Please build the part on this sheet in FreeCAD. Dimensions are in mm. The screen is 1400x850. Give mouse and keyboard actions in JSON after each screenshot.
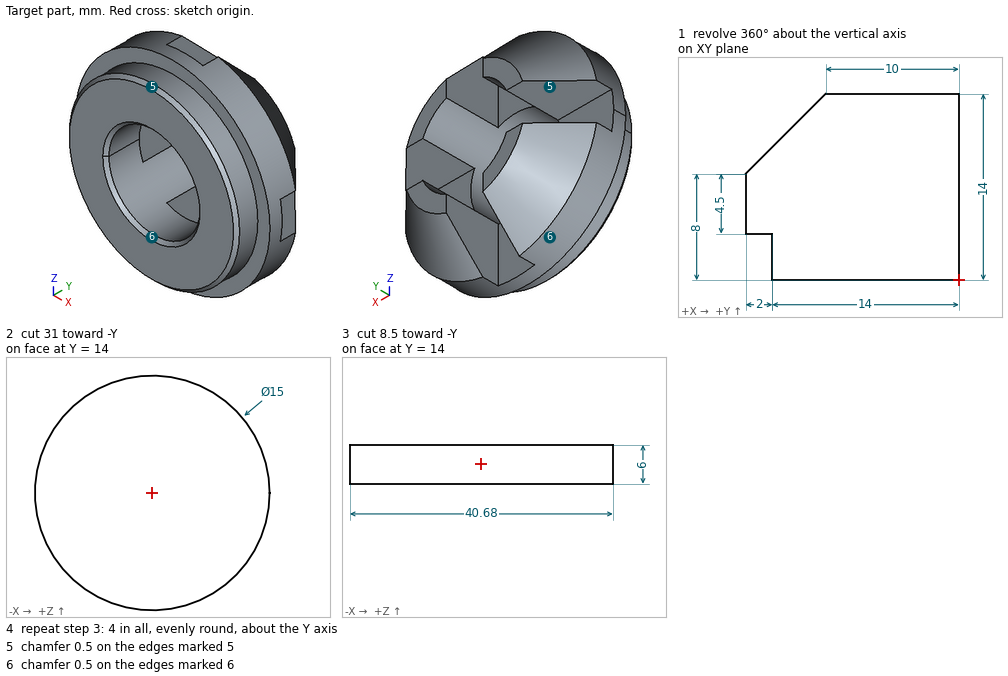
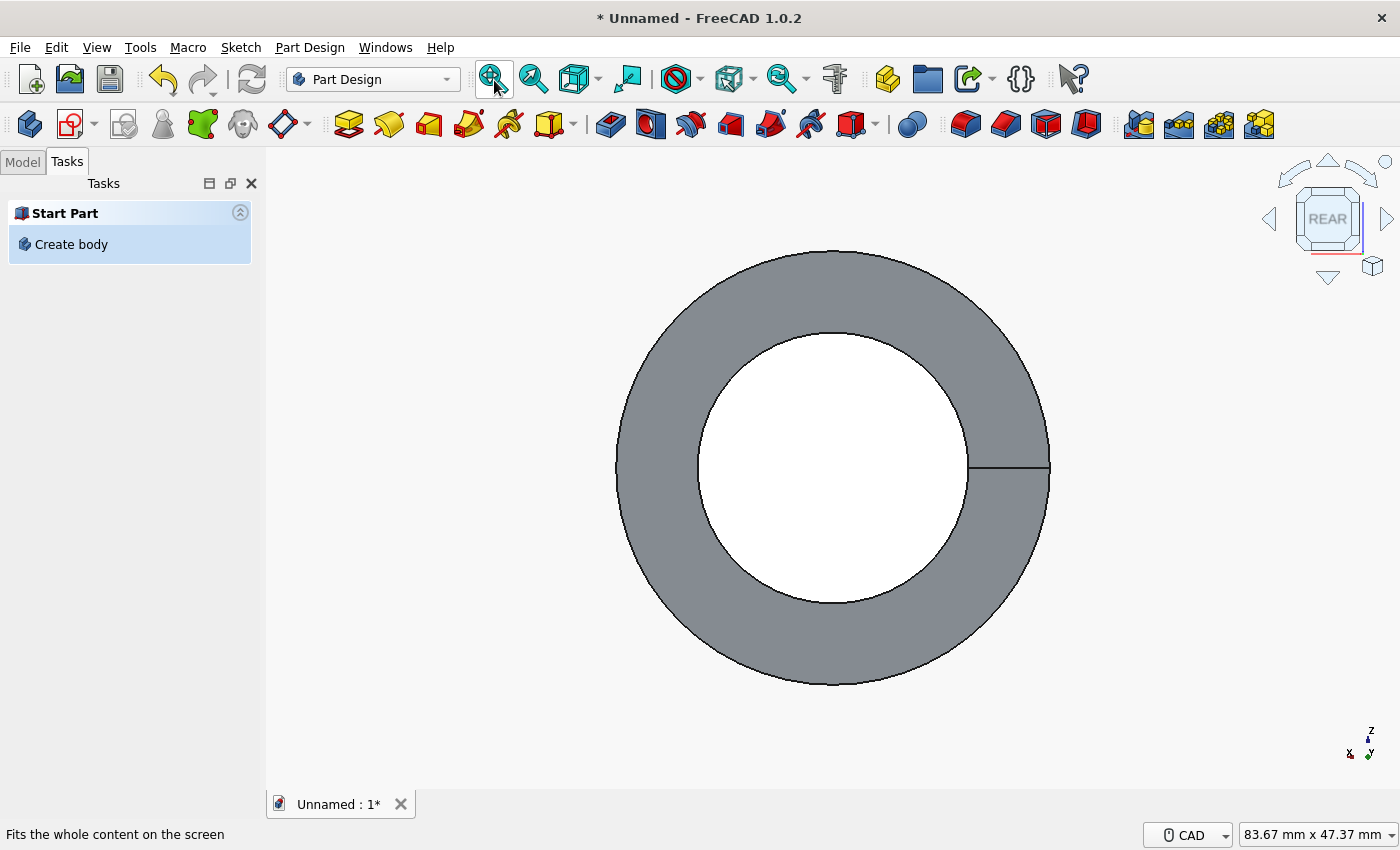
{"action": "left_click", "coordinate": [833, 467]}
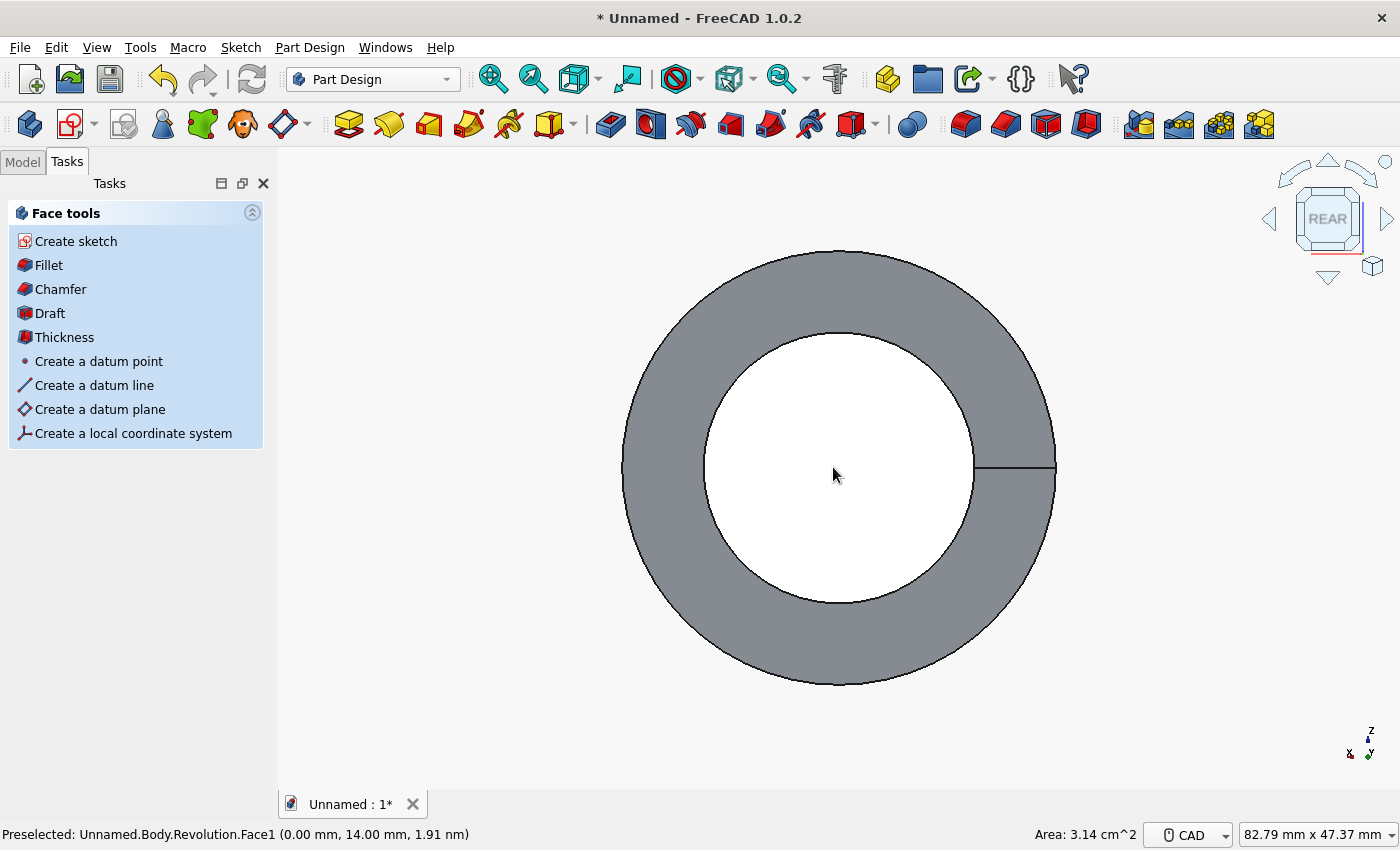
{"action": "left_click", "coordinate": [70, 124]}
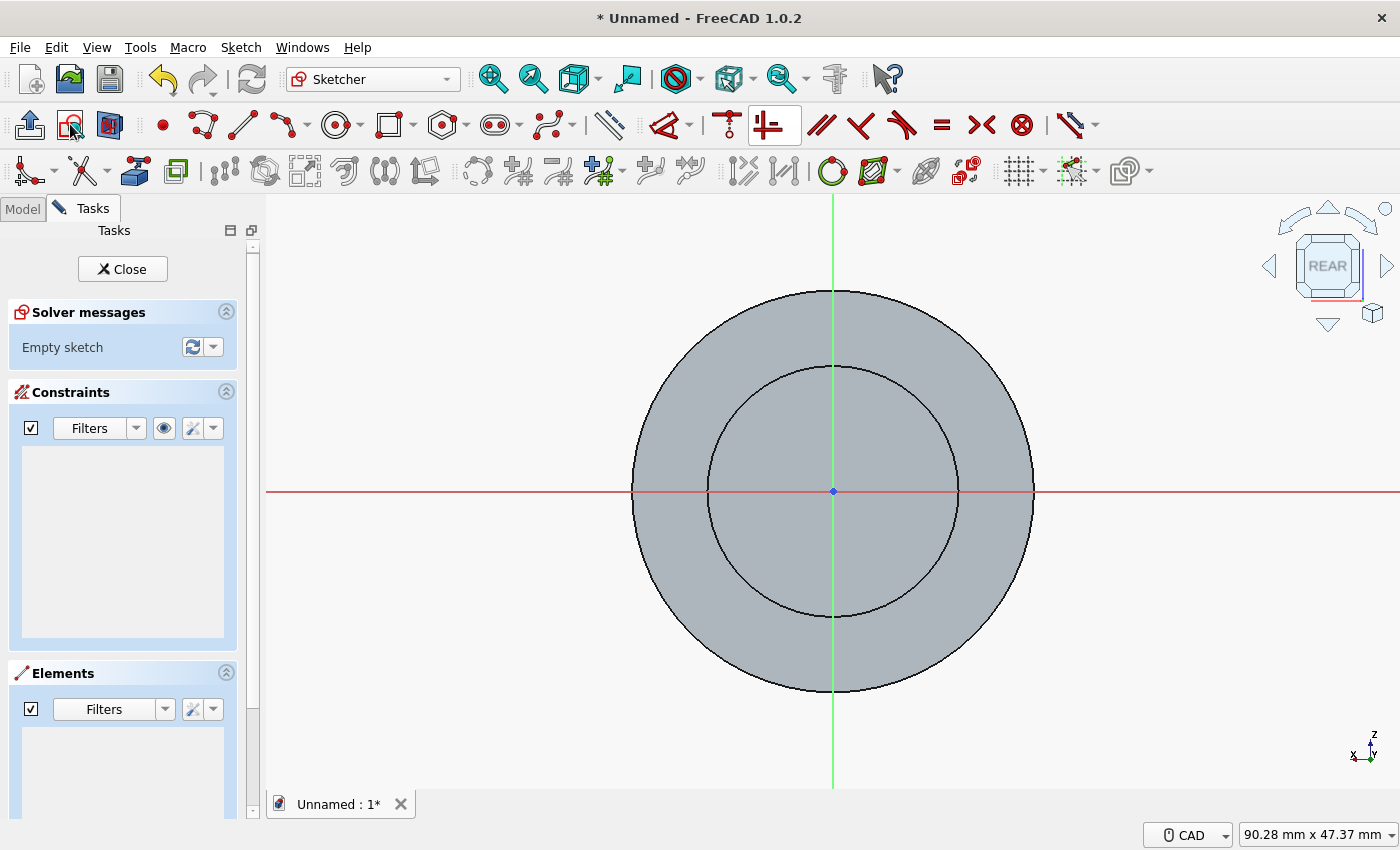
{"action": "scroll", "coordinate": [889, 492], "scroll_direction": "up", "scroll_amount": 4}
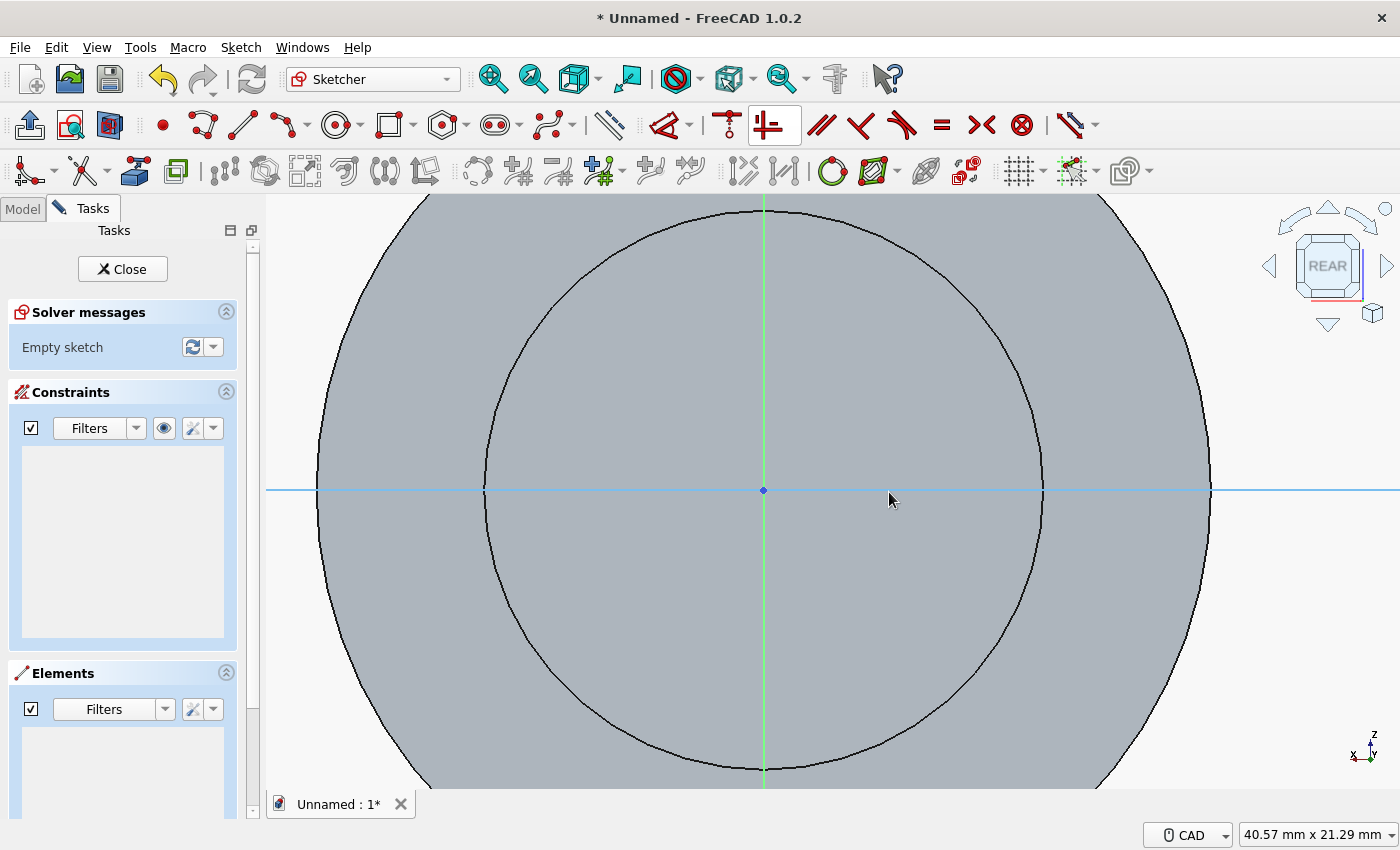
{"action": "left_click", "coordinate": [336, 126]}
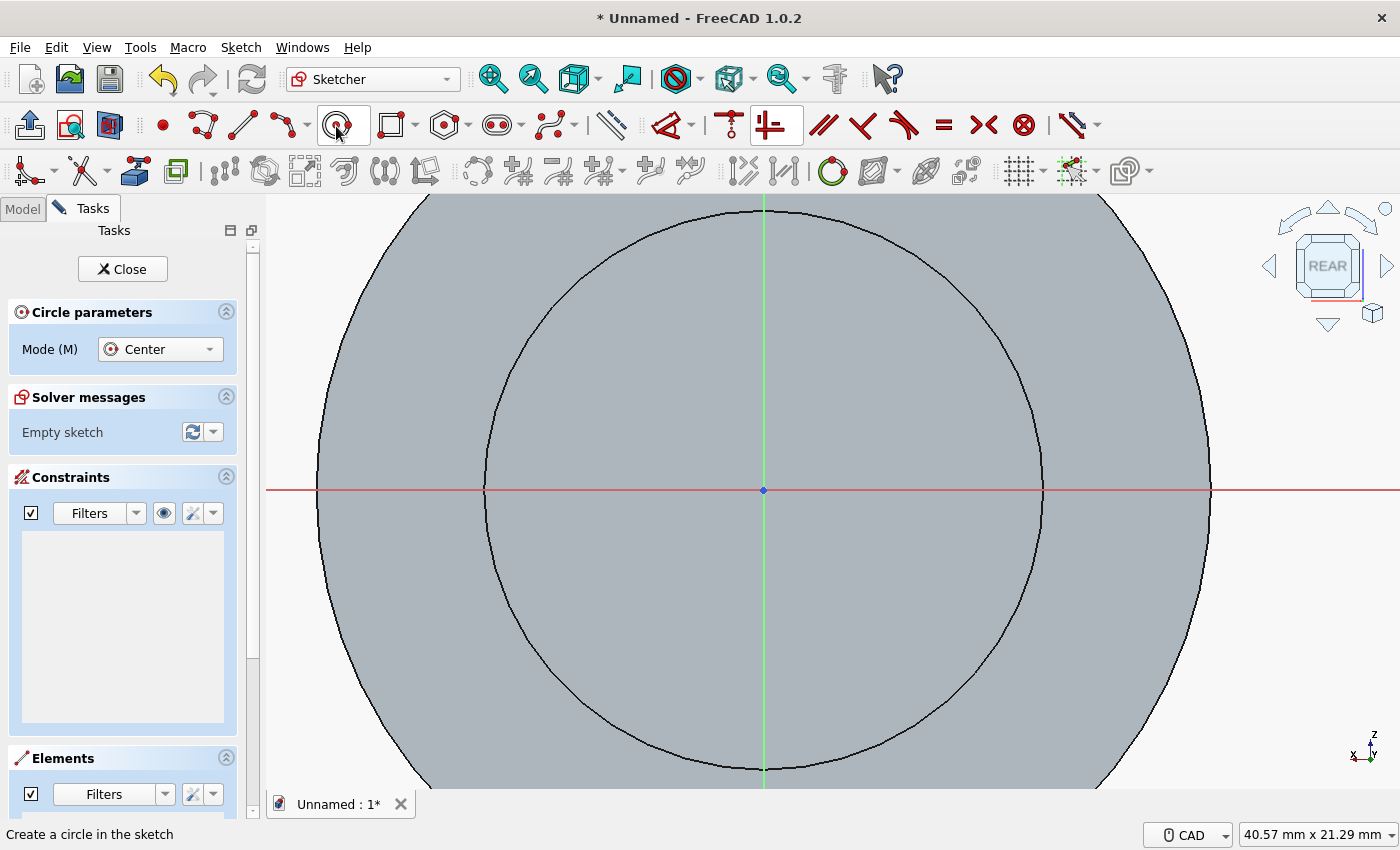
{"action": "left_click", "coordinate": [764, 490]}
{"action": "left_click", "coordinate": [912, 342]}
{"action": "key", "text": "Escape"}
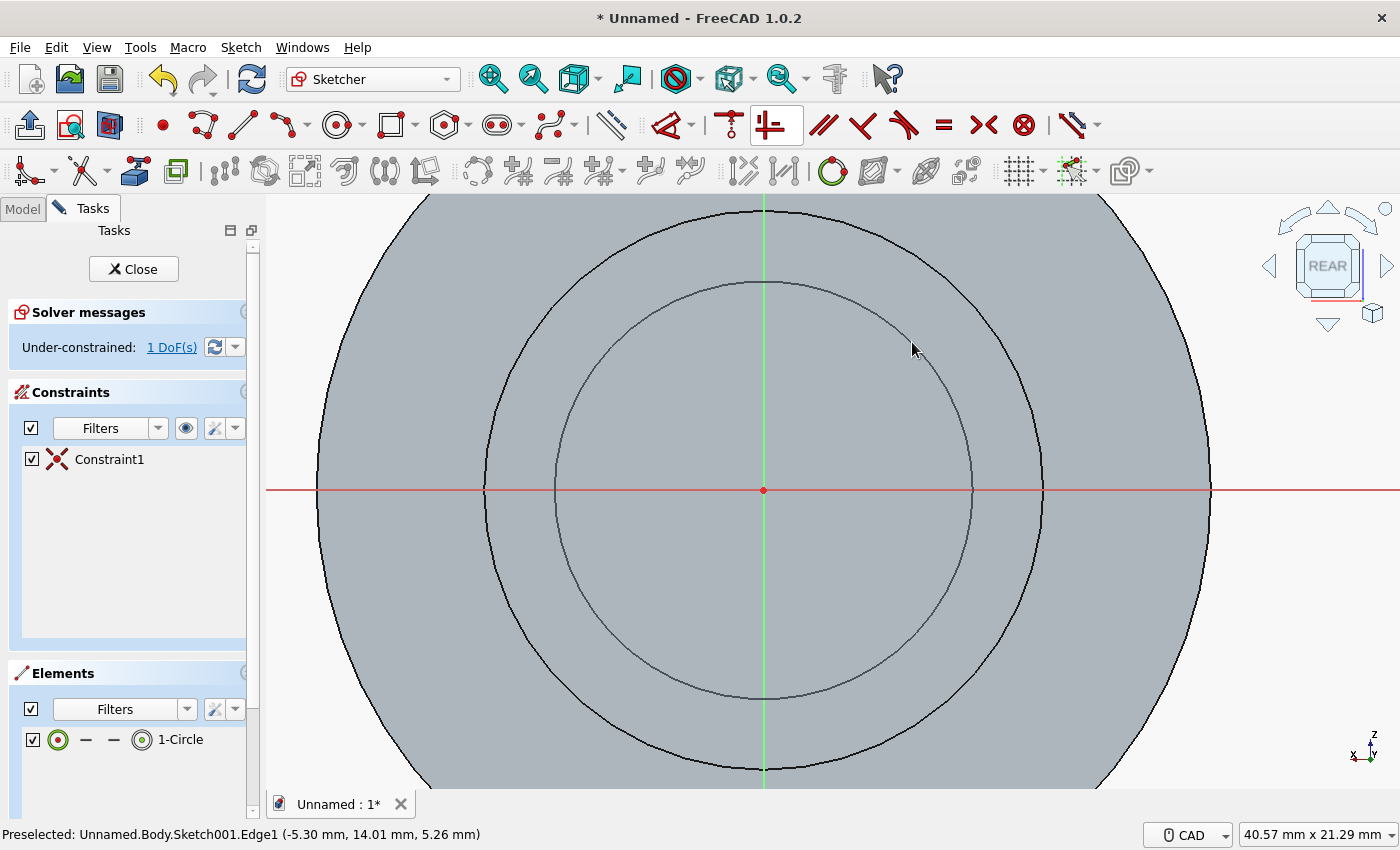
{"action": "left_click", "coordinate": [666, 126]}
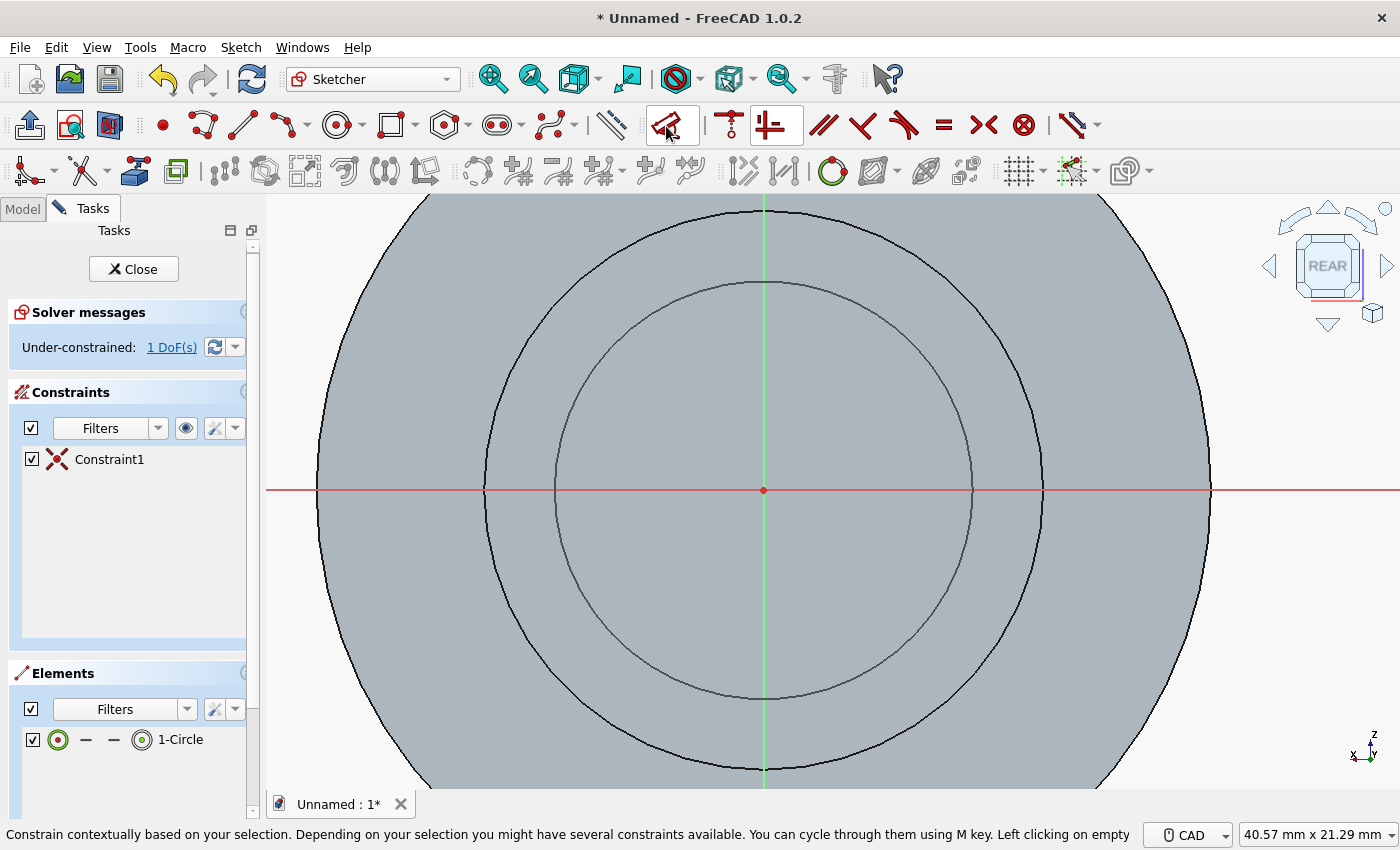
{"action": "left_click", "coordinate": [911, 342]}
{"action": "left_click", "coordinate": [934, 319]}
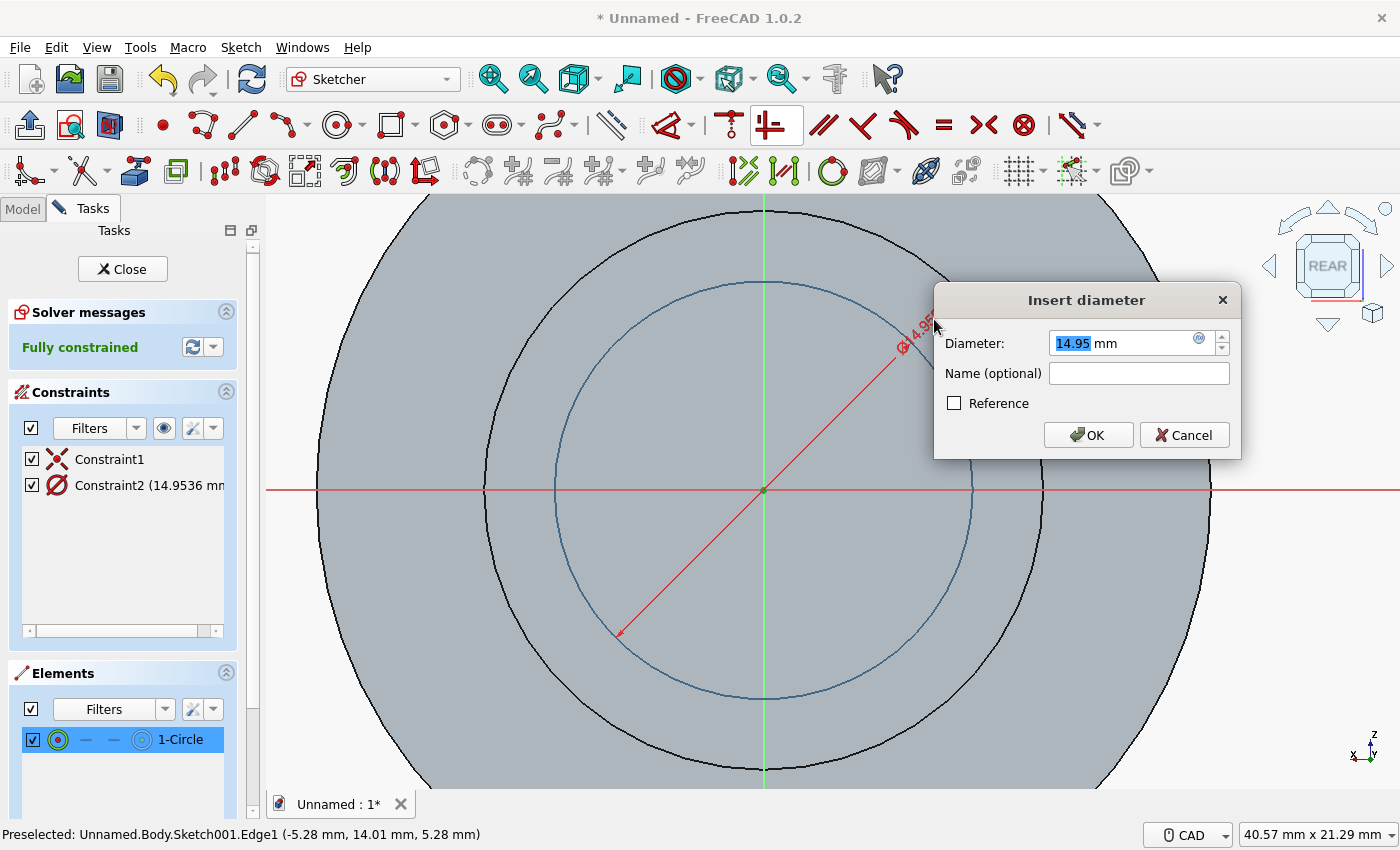
{"action": "type", "text": "15"}
{"action": "key", "text": "Return"}
{"action": "key", "text": "Escape"}